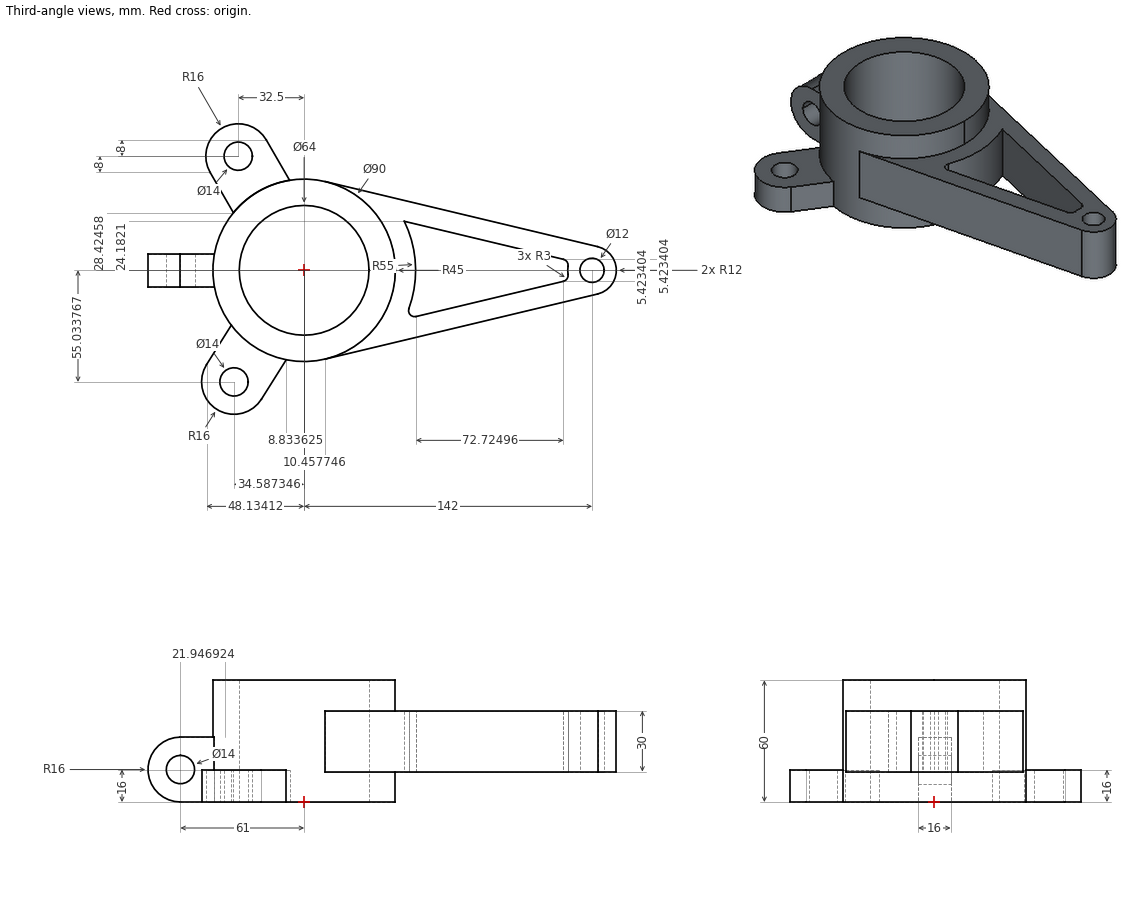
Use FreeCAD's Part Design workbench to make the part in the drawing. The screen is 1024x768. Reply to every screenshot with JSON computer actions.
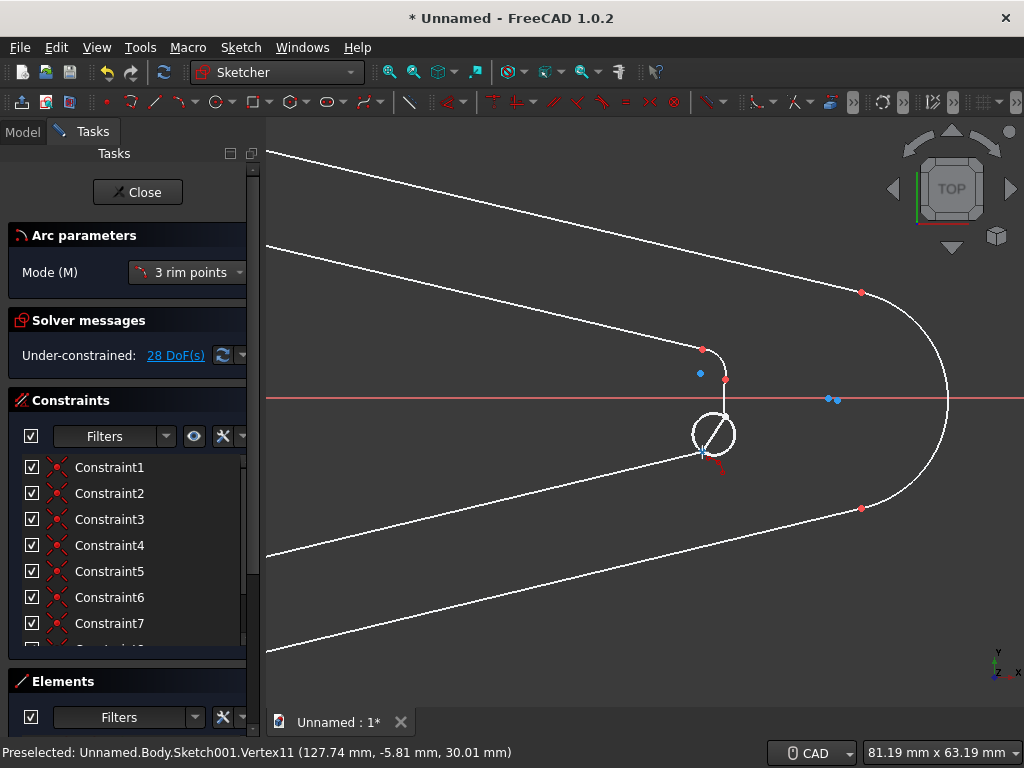
{"action": "scroll", "coordinate": [721, 437], "scroll_direction": "up", "scroll_amount": 4}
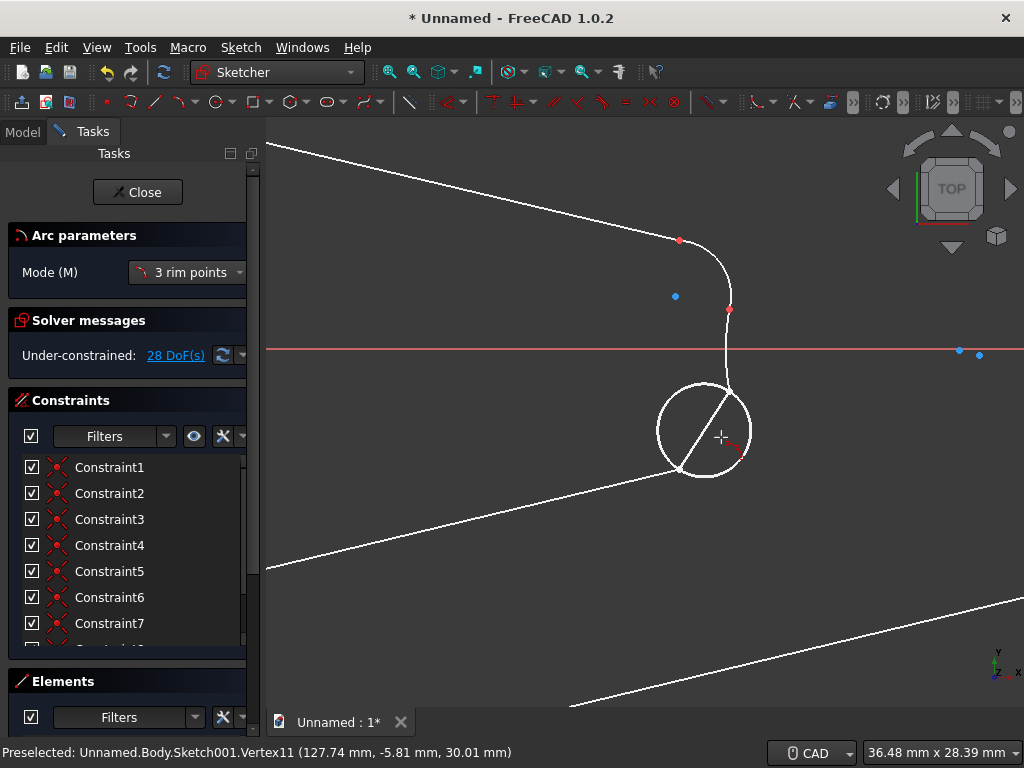
{"action": "left_click", "coordinate": [720, 435]}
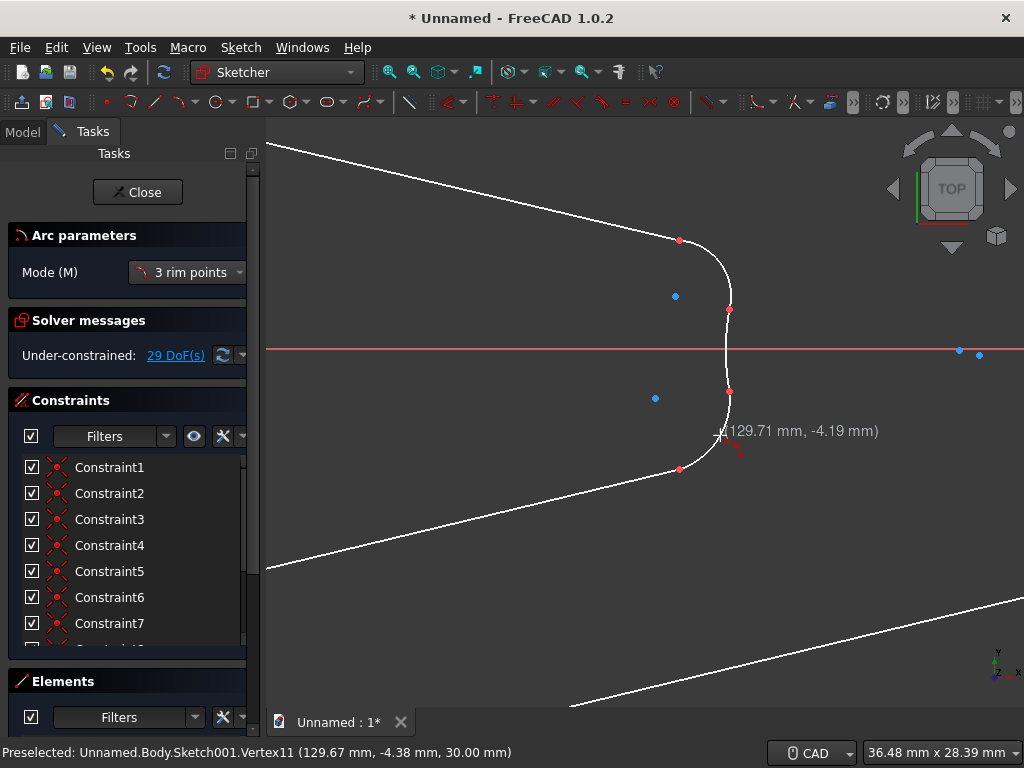
{"action": "key", "text": "g c"}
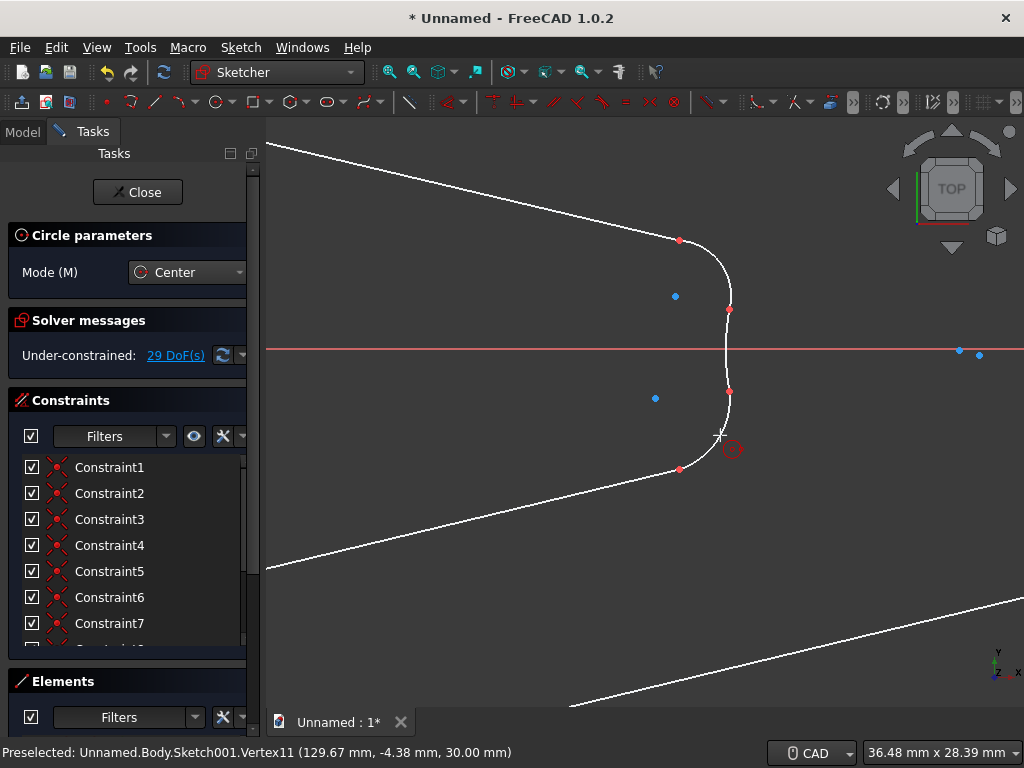
{"action": "scroll", "coordinate": [725, 422], "scroll_direction": "down", "scroll_amount": 10}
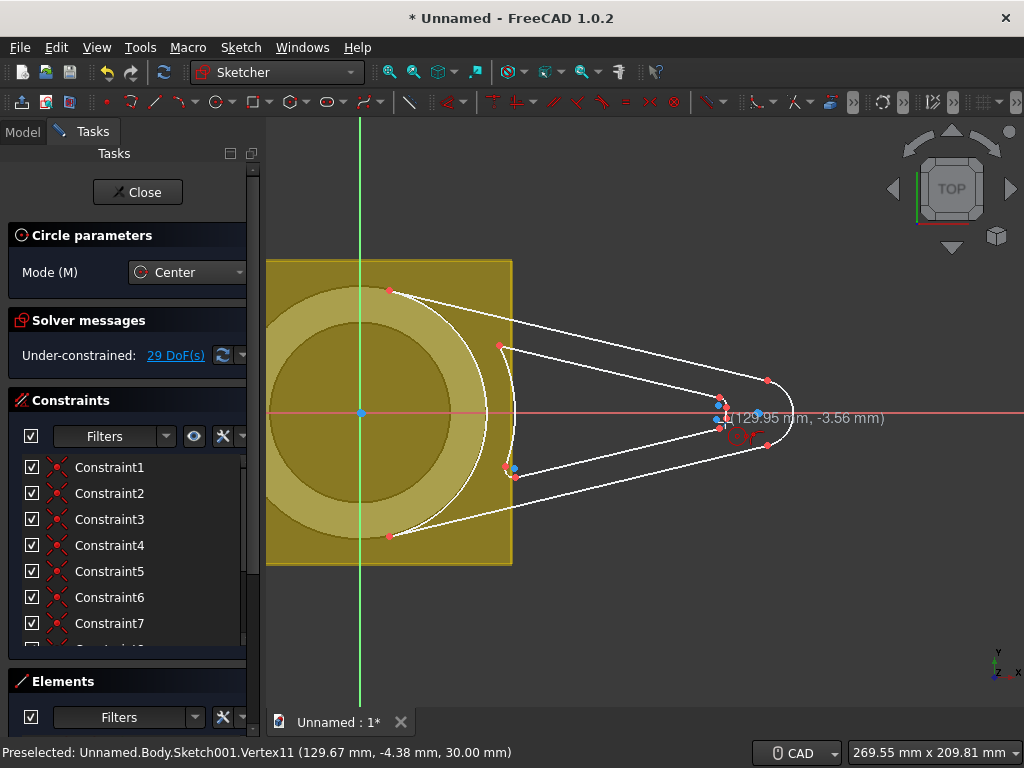
{"action": "scroll", "coordinate": [759, 413], "scroll_direction": "up", "scroll_amount": 2}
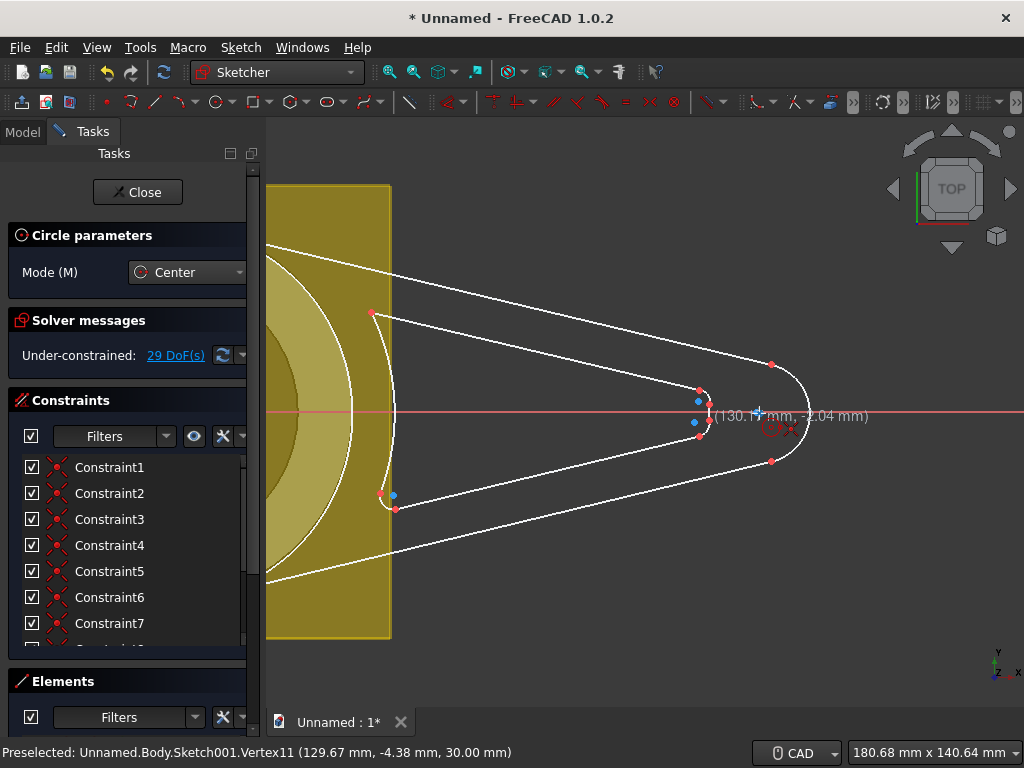
{"action": "left_click", "coordinate": [759, 412]}
{"action": "left_click", "coordinate": [777, 394]}
{"action": "key", "text": "Escape"}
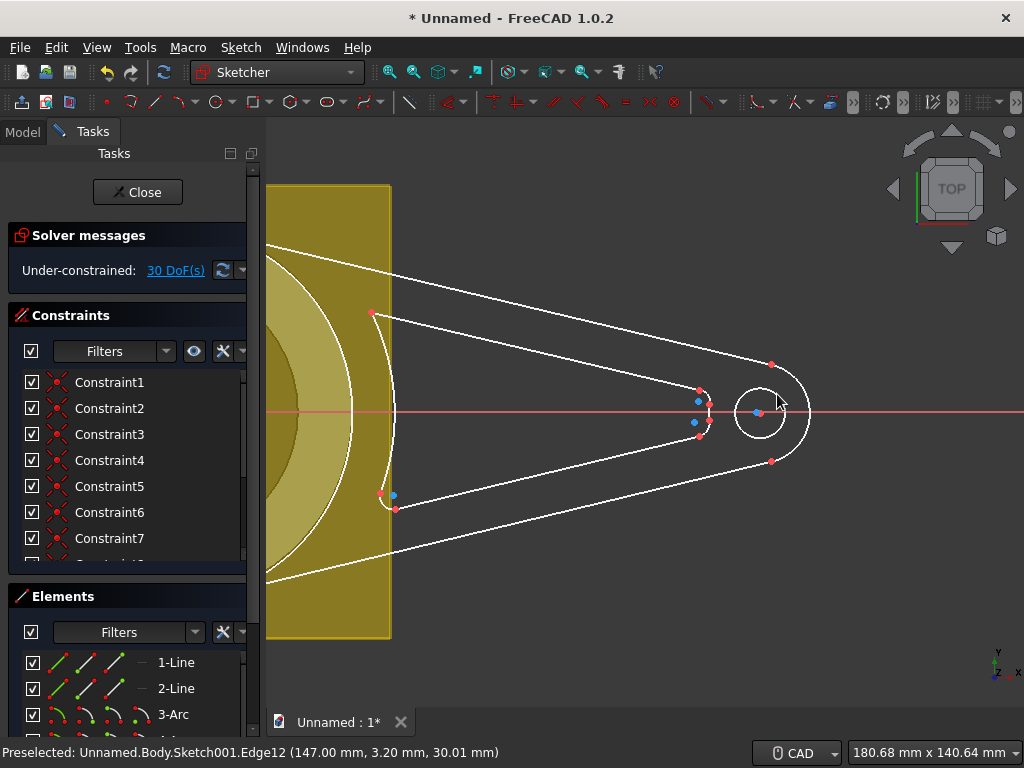
{"action": "left_click", "coordinate": [376, 557]}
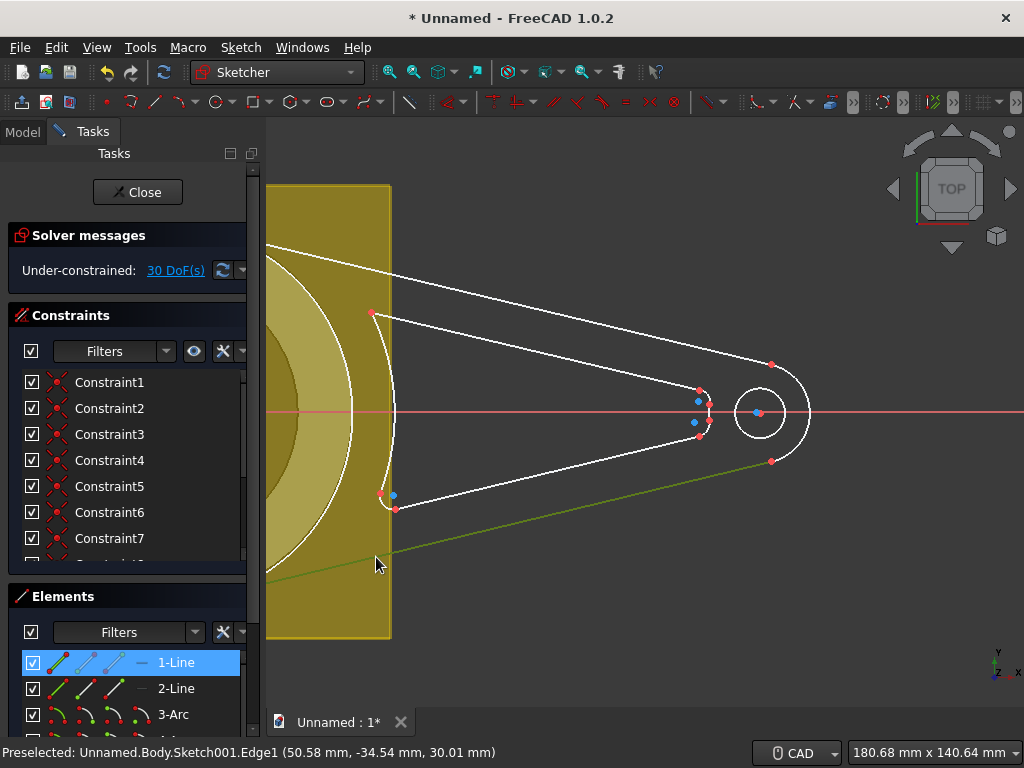
{"action": "left_click", "coordinate": [803, 439]}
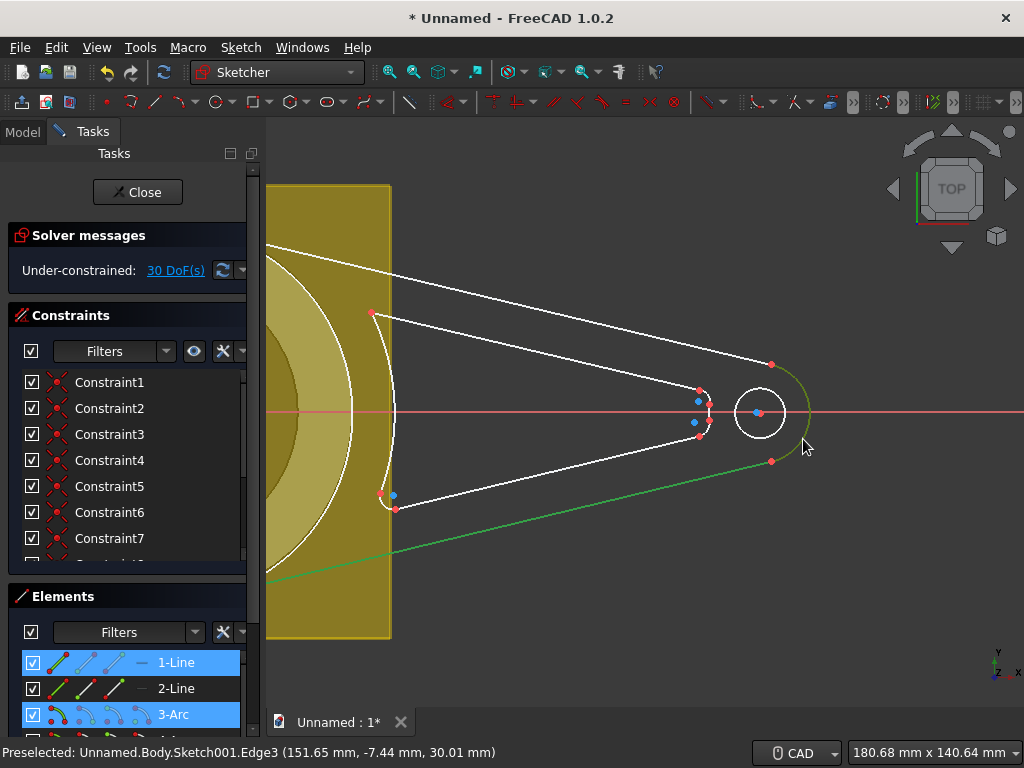
{"action": "key", "text": "t"}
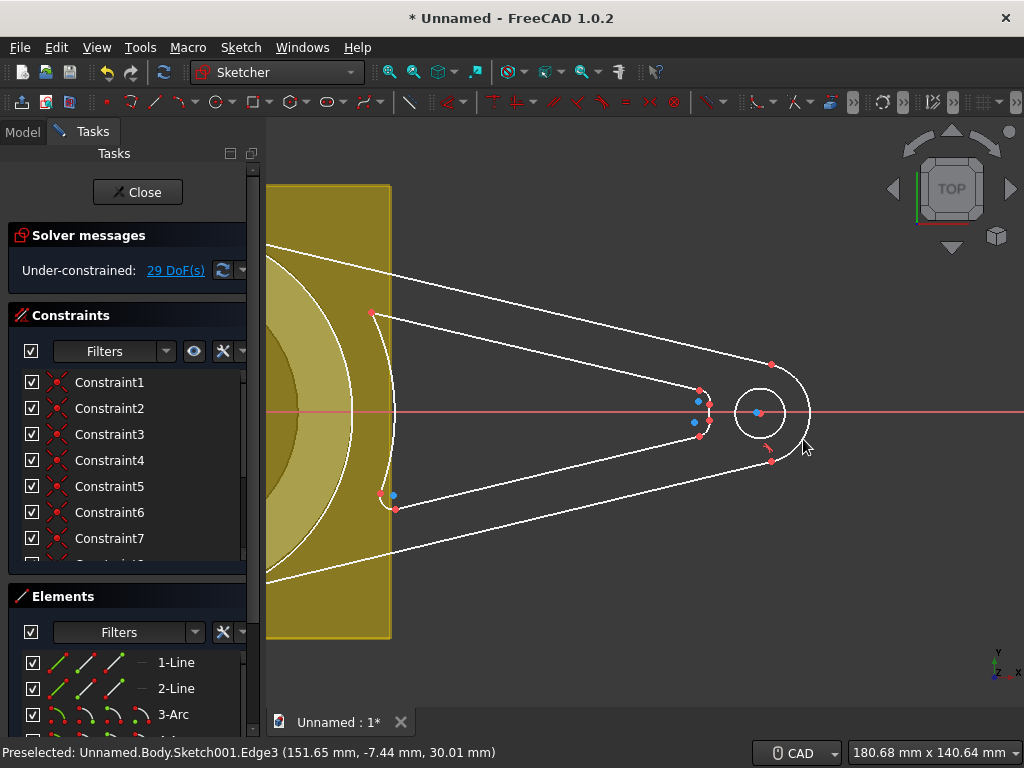
{"action": "left_click", "coordinate": [602, 325]}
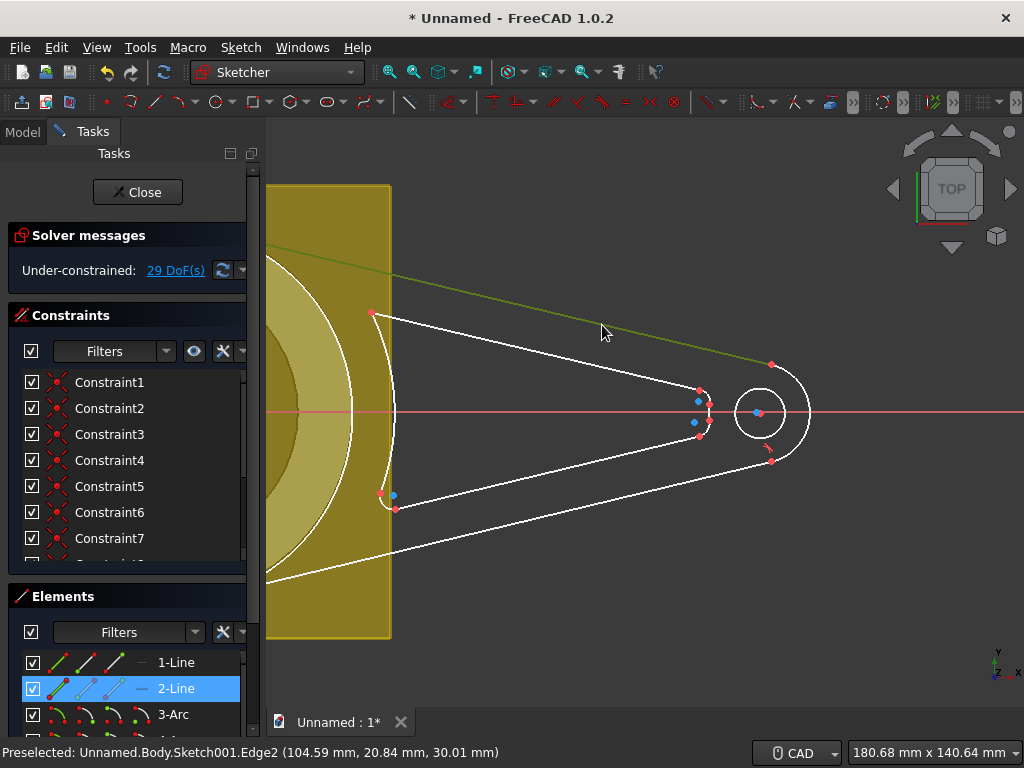
{"action": "left_click", "coordinate": [803, 439]}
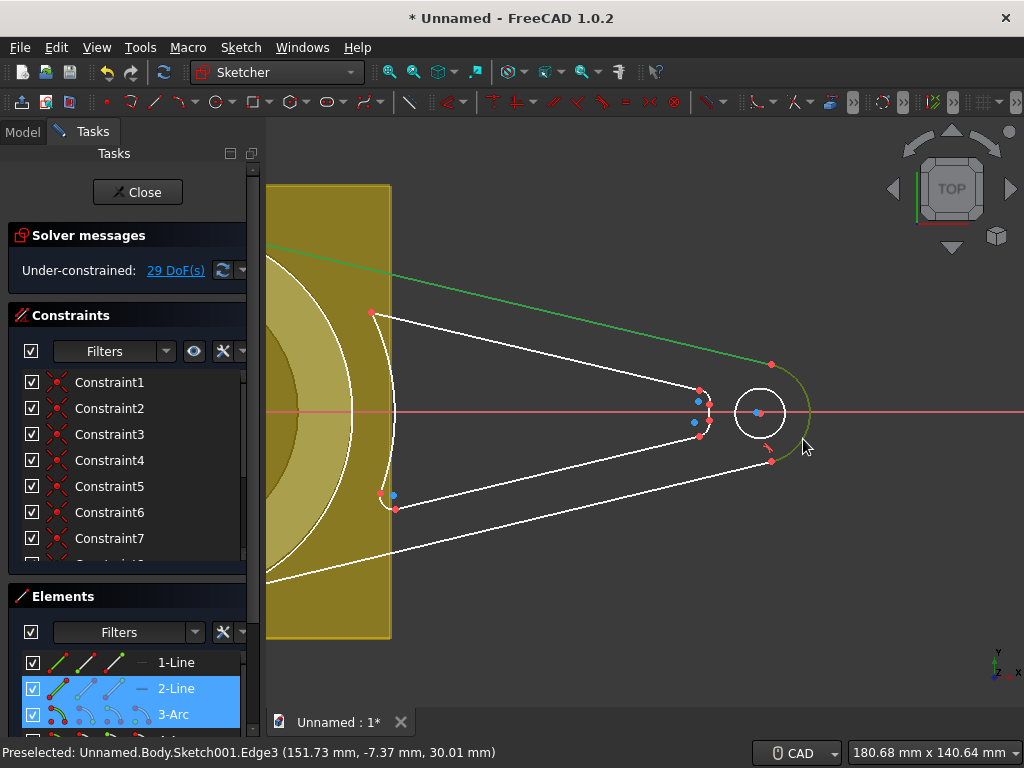
{"action": "key", "text": "t"}